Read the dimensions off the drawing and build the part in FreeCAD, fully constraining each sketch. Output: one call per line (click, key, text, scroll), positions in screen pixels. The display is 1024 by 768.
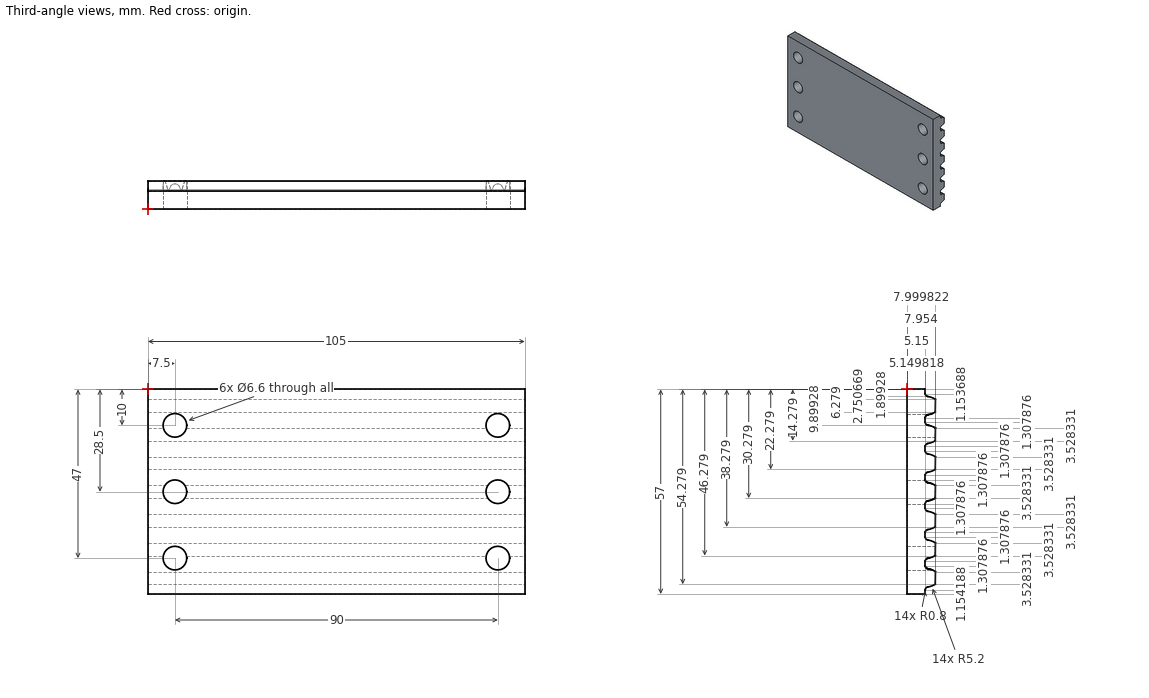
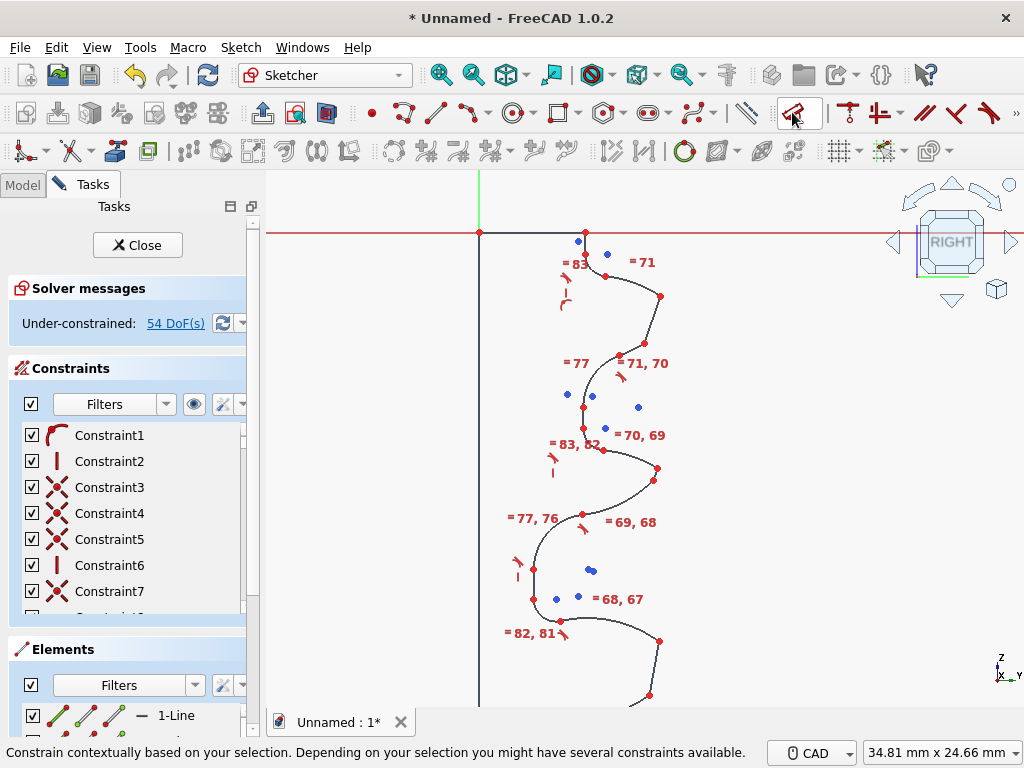
scroll(581, 260, down, 6)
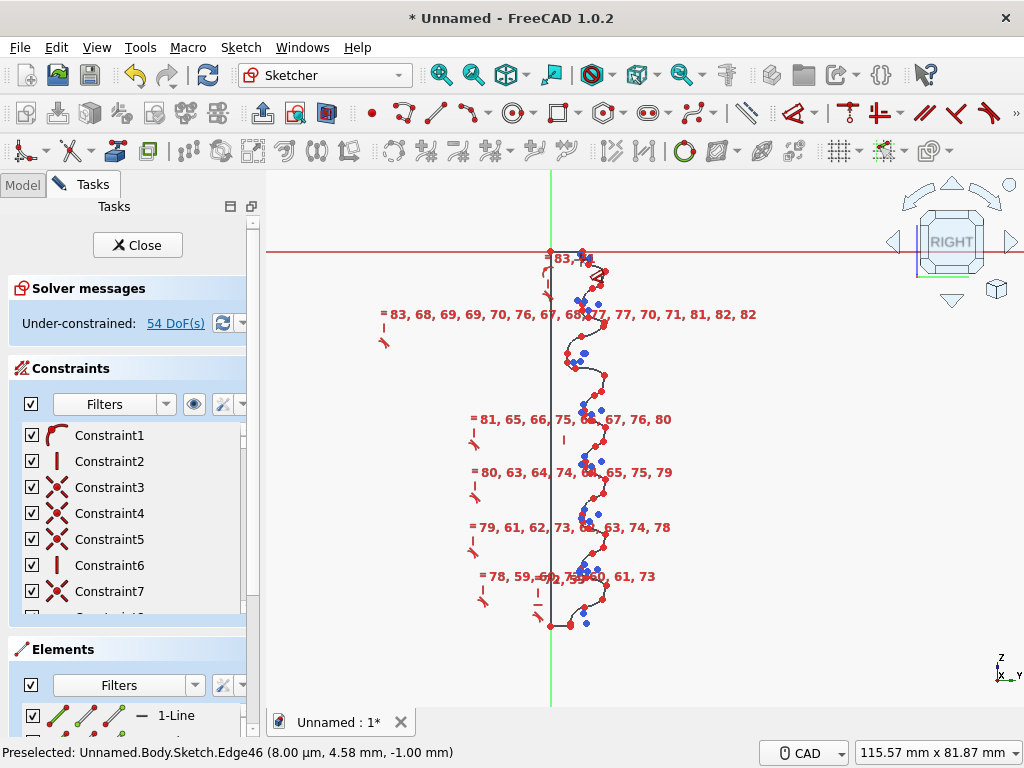
scroll(578, 610, up, 11)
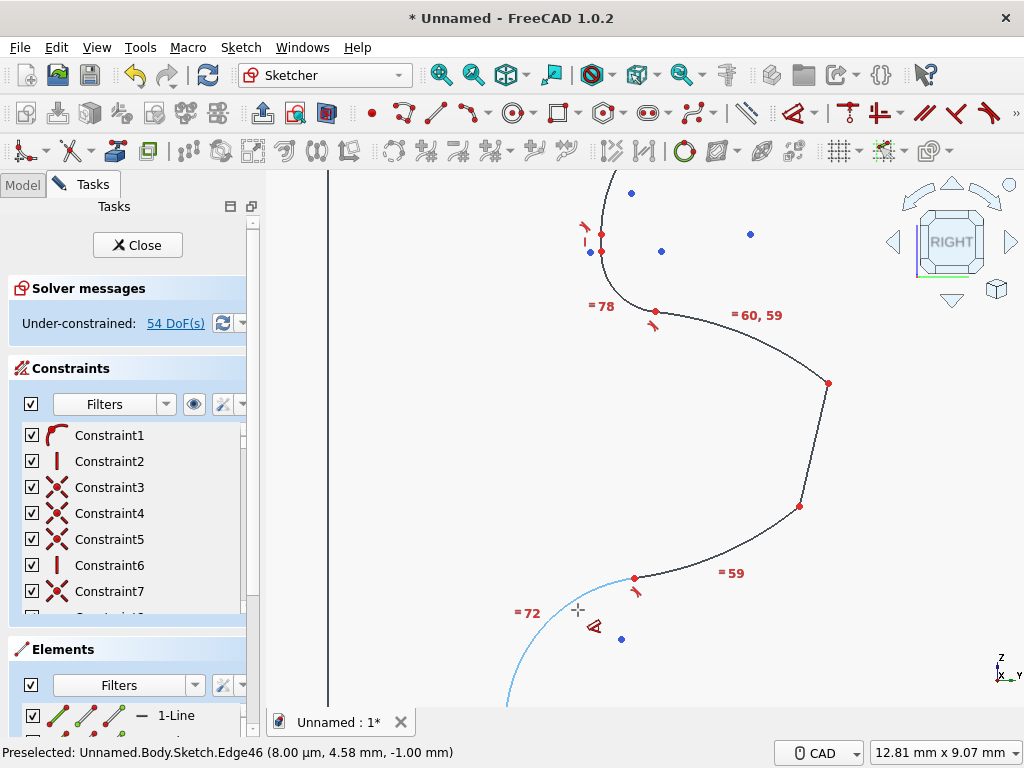
click(575, 600)
click(558, 573)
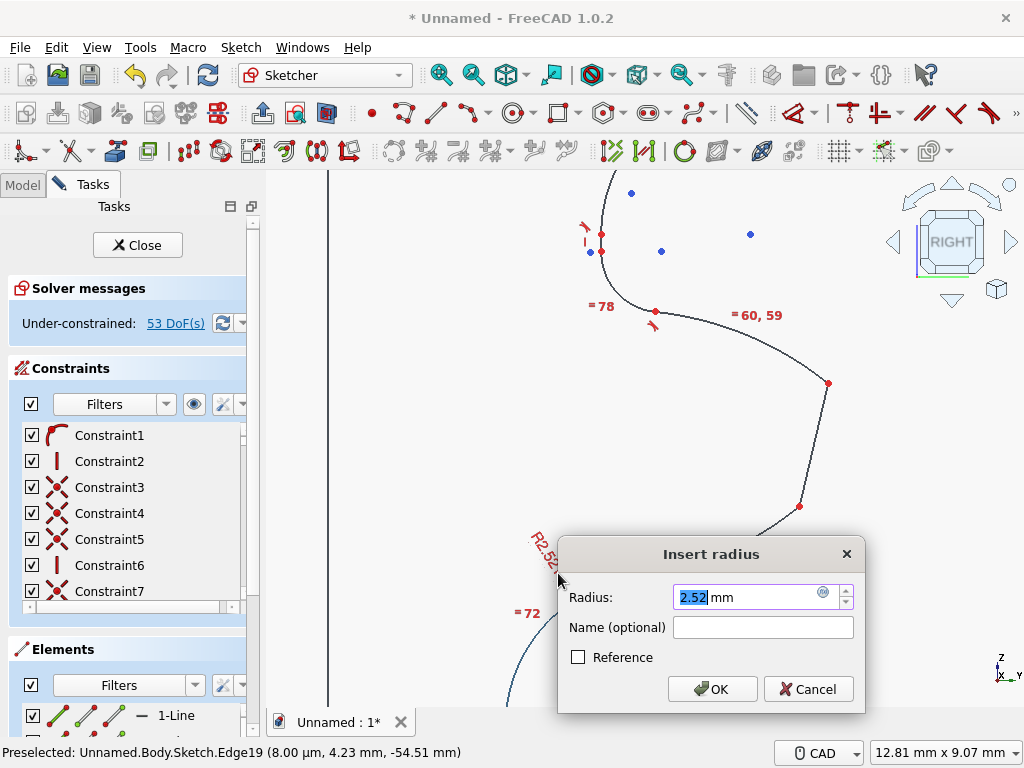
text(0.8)
key(Return)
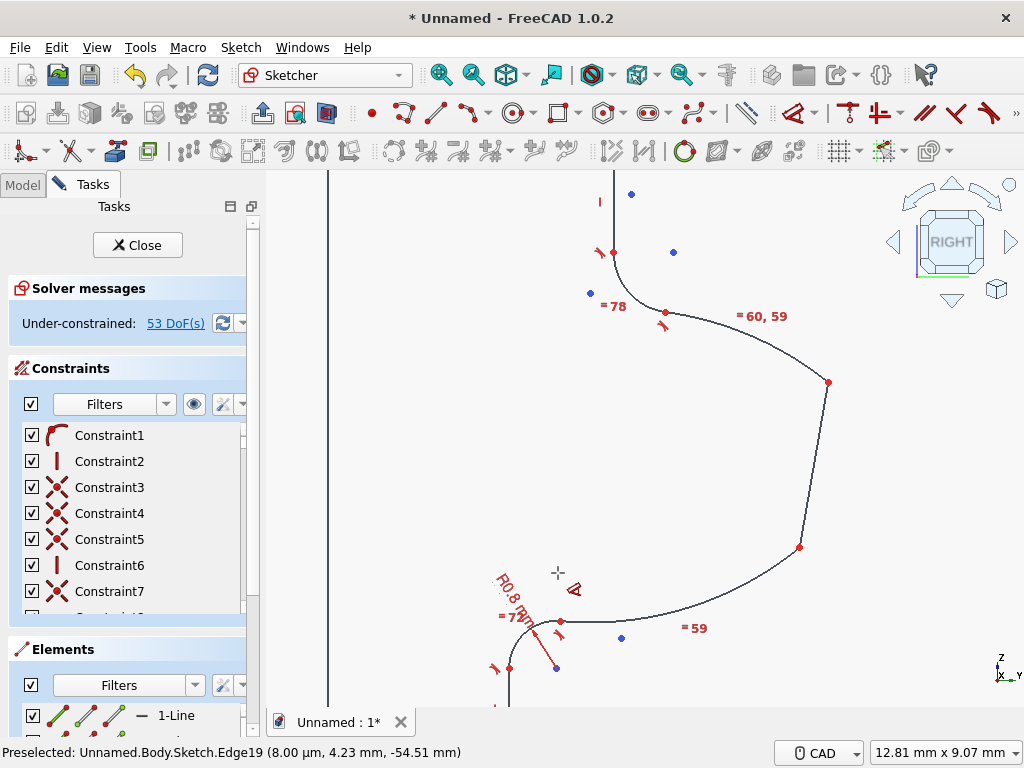
scroll(578, 610, down, 11)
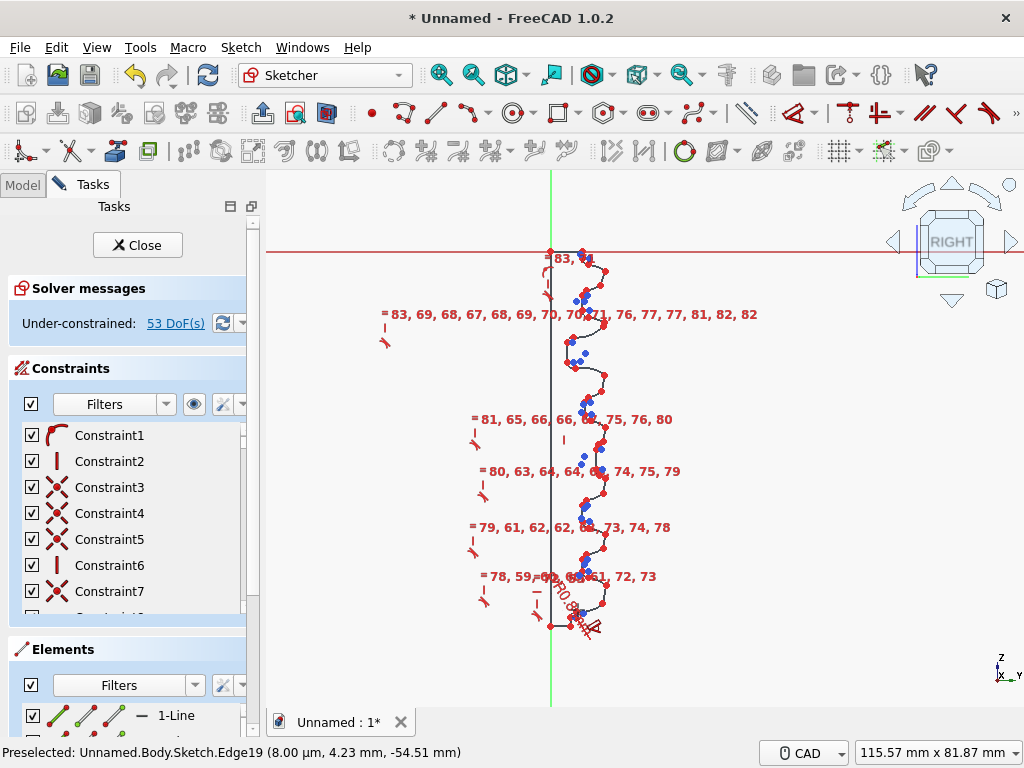
scroll(585, 612, up, 3)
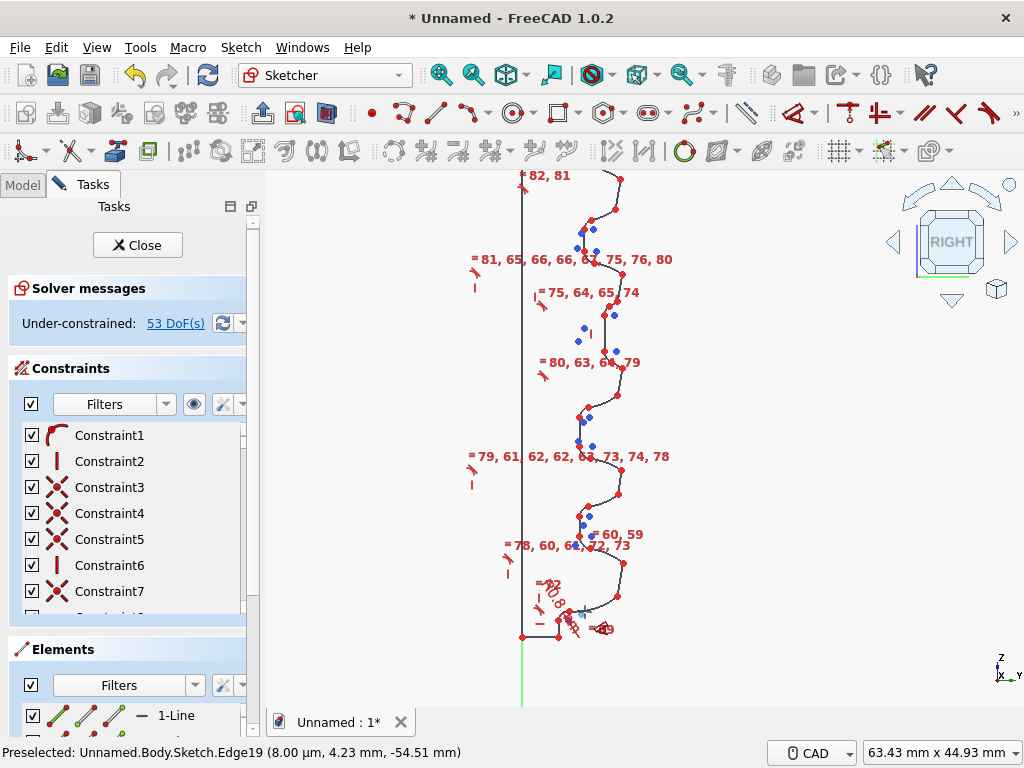
click(604, 605)
click(618, 634)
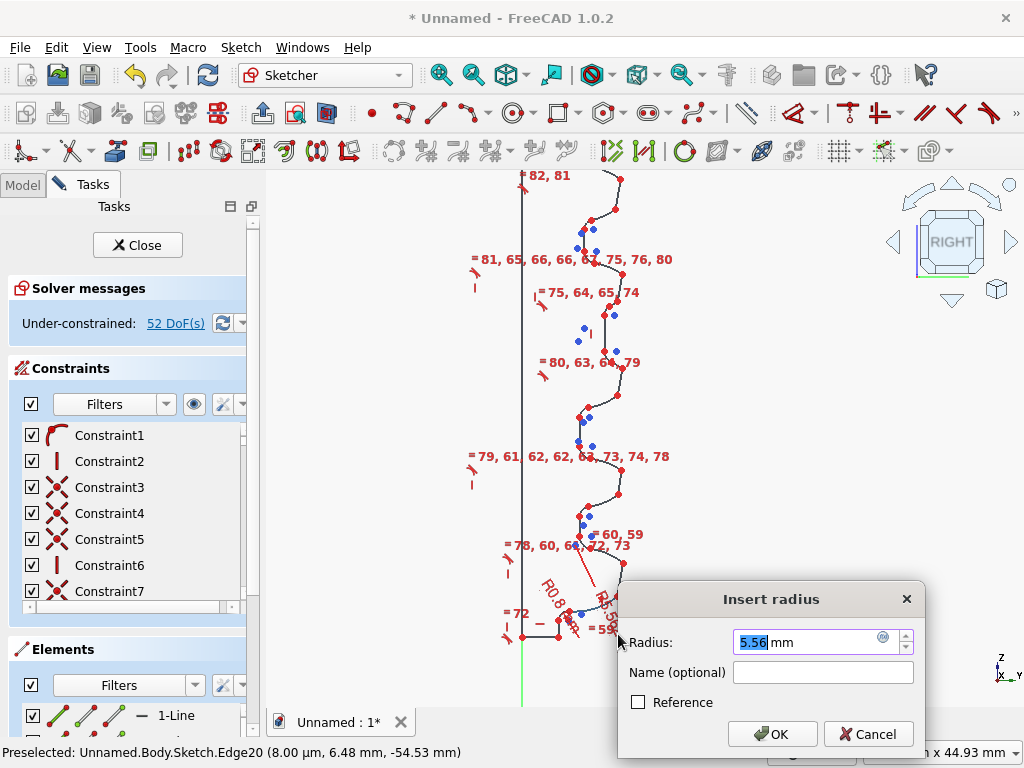
text(5.2)
key(Return)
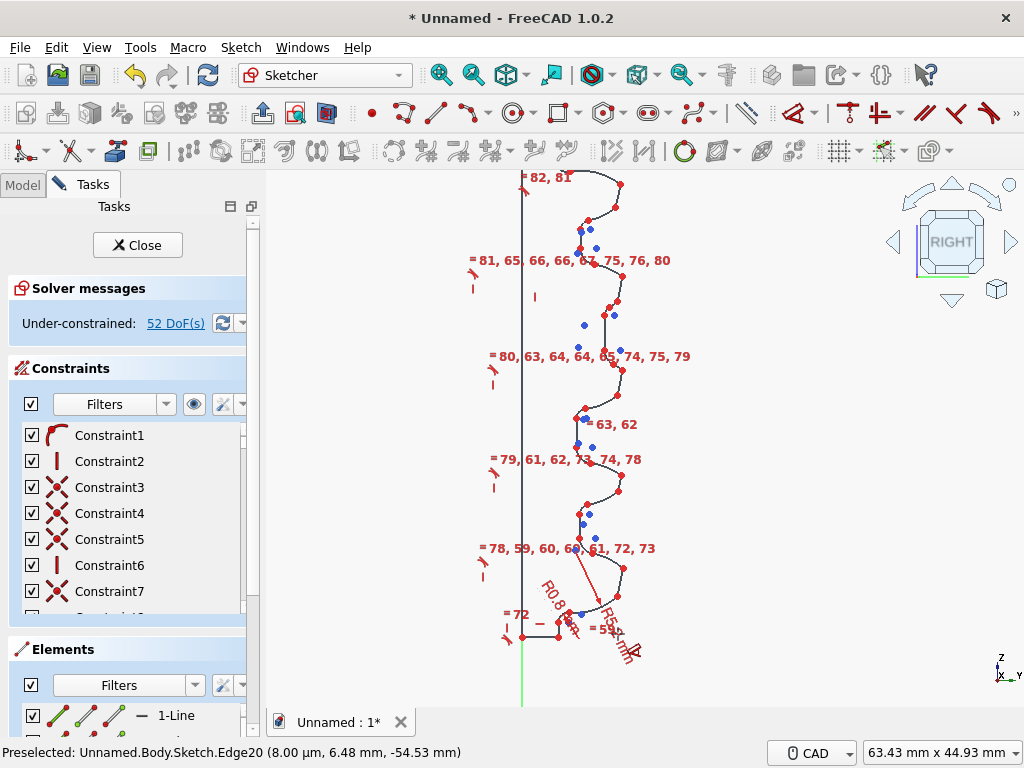
scroll(583, 548, up, 8)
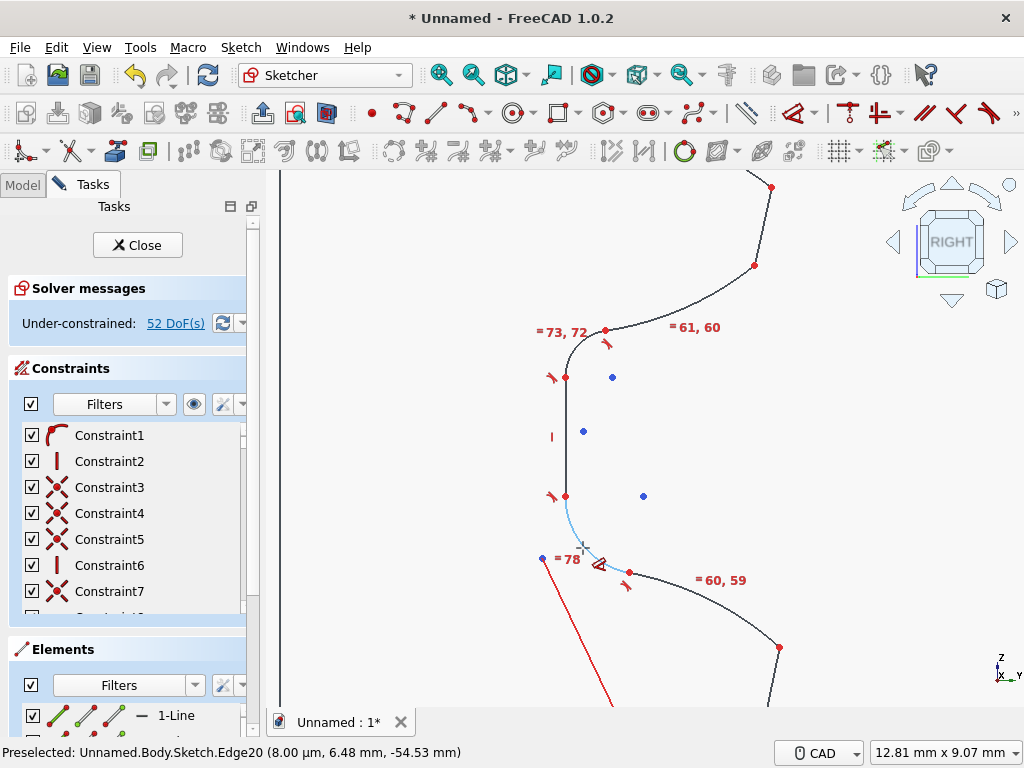
click(583, 546)
click(558, 566)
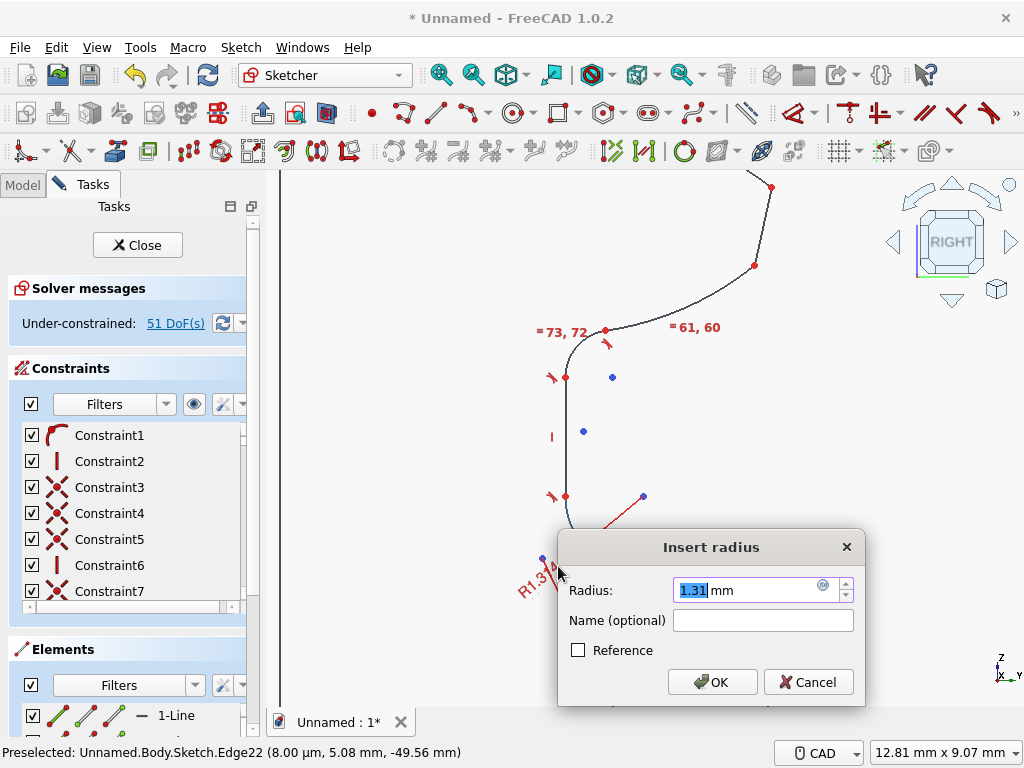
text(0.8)
key(Return)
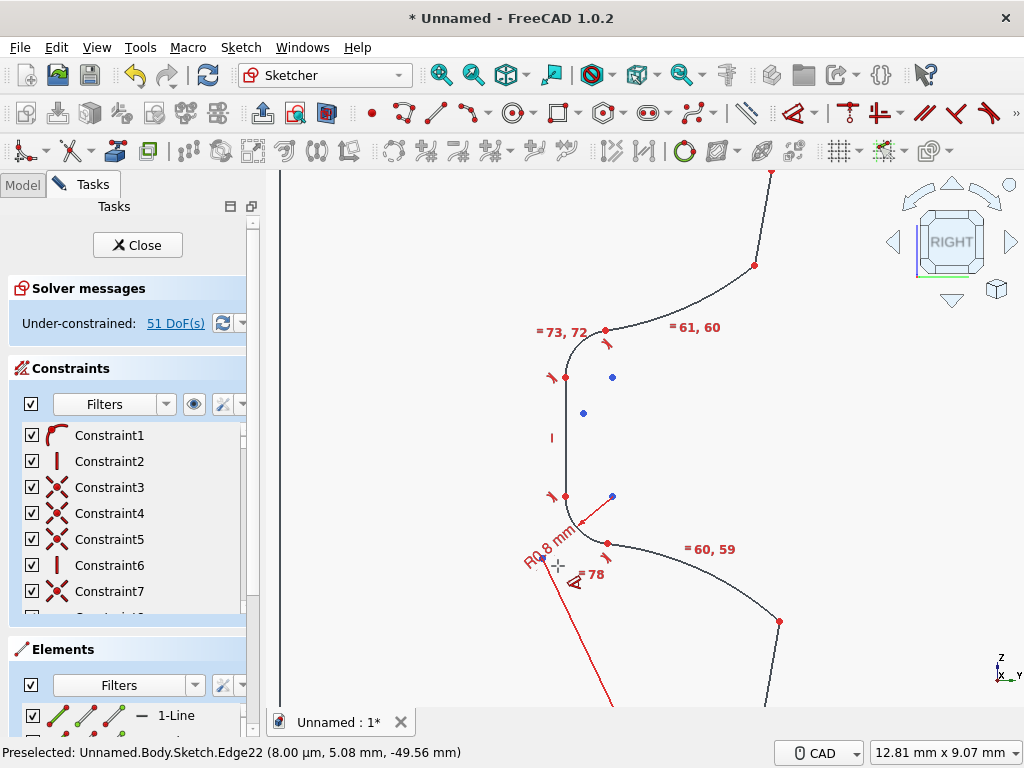
scroll(584, 581, down, 11)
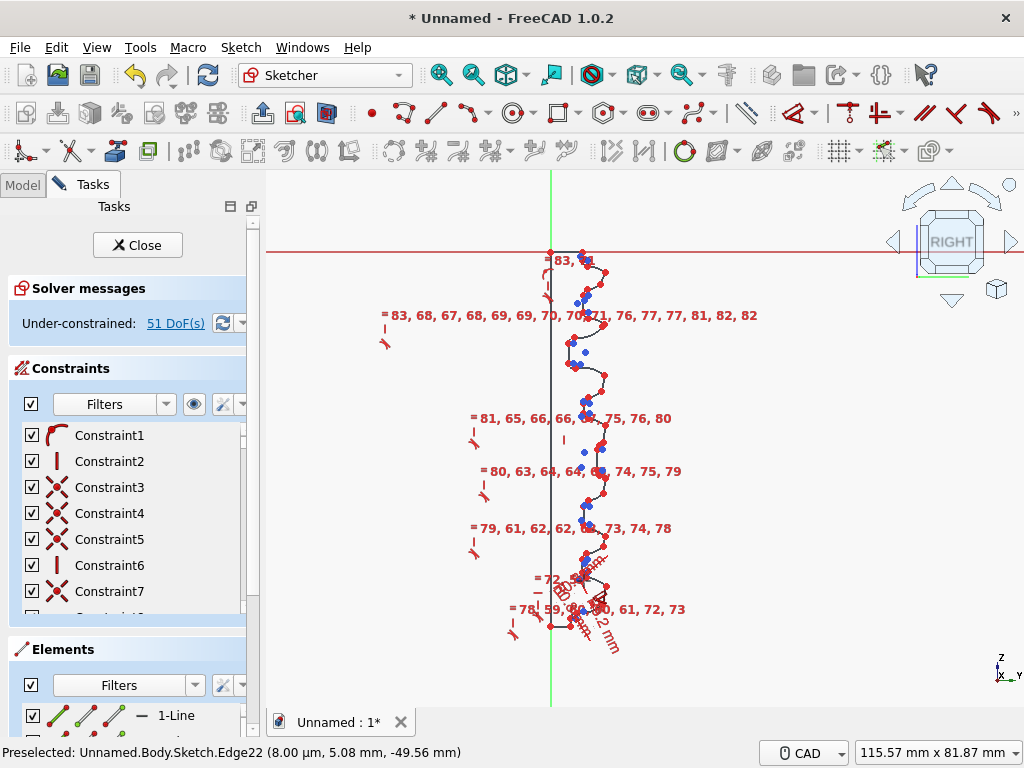
click(551, 365)
click(517, 440)